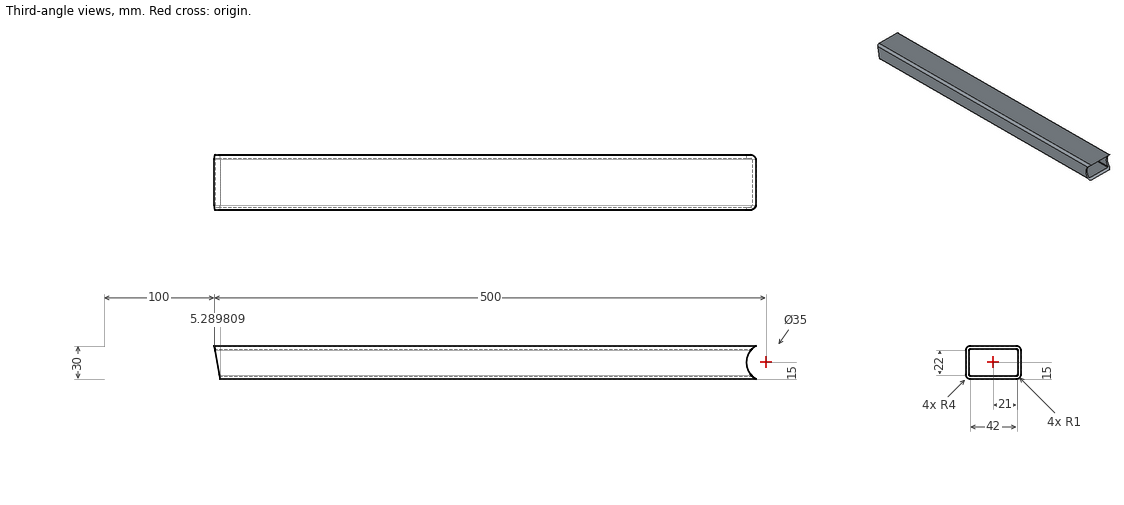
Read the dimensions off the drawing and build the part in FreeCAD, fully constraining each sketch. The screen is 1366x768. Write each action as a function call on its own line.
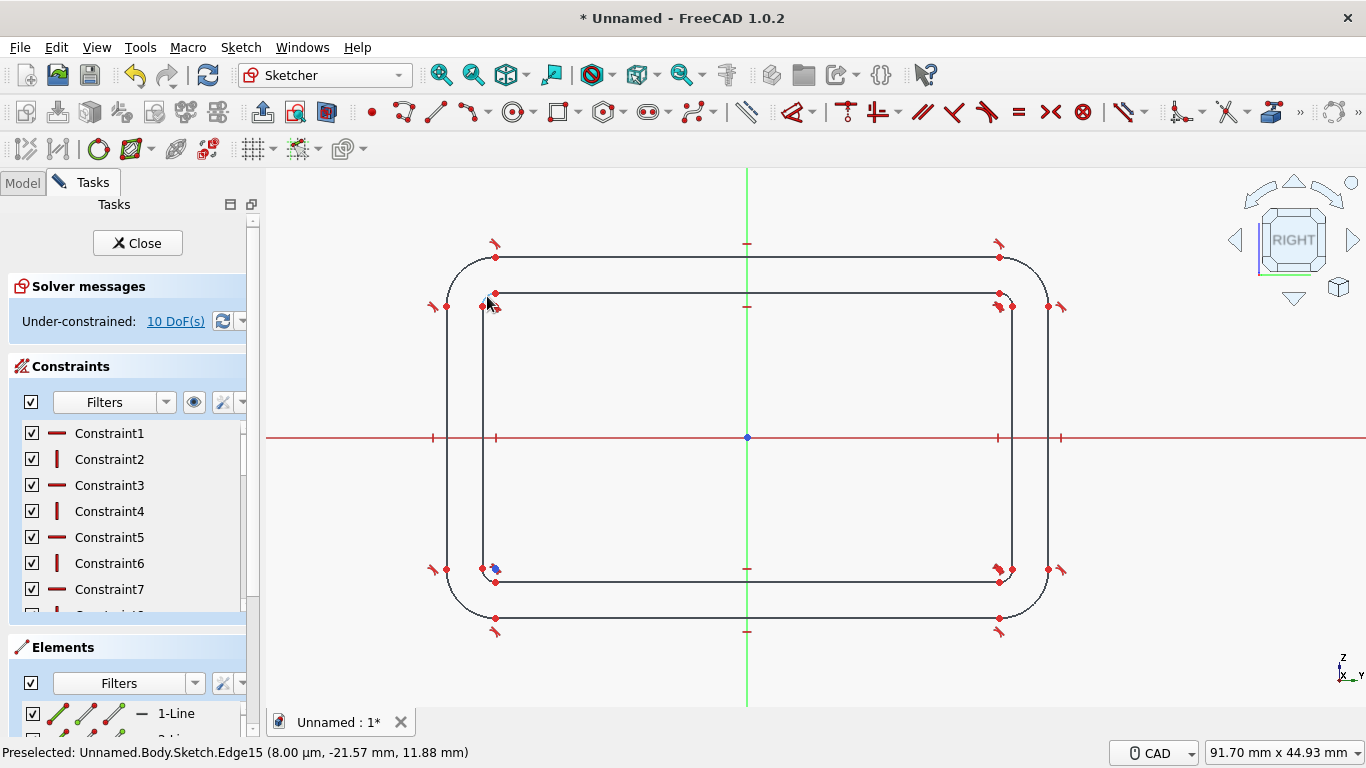
click(452, 591)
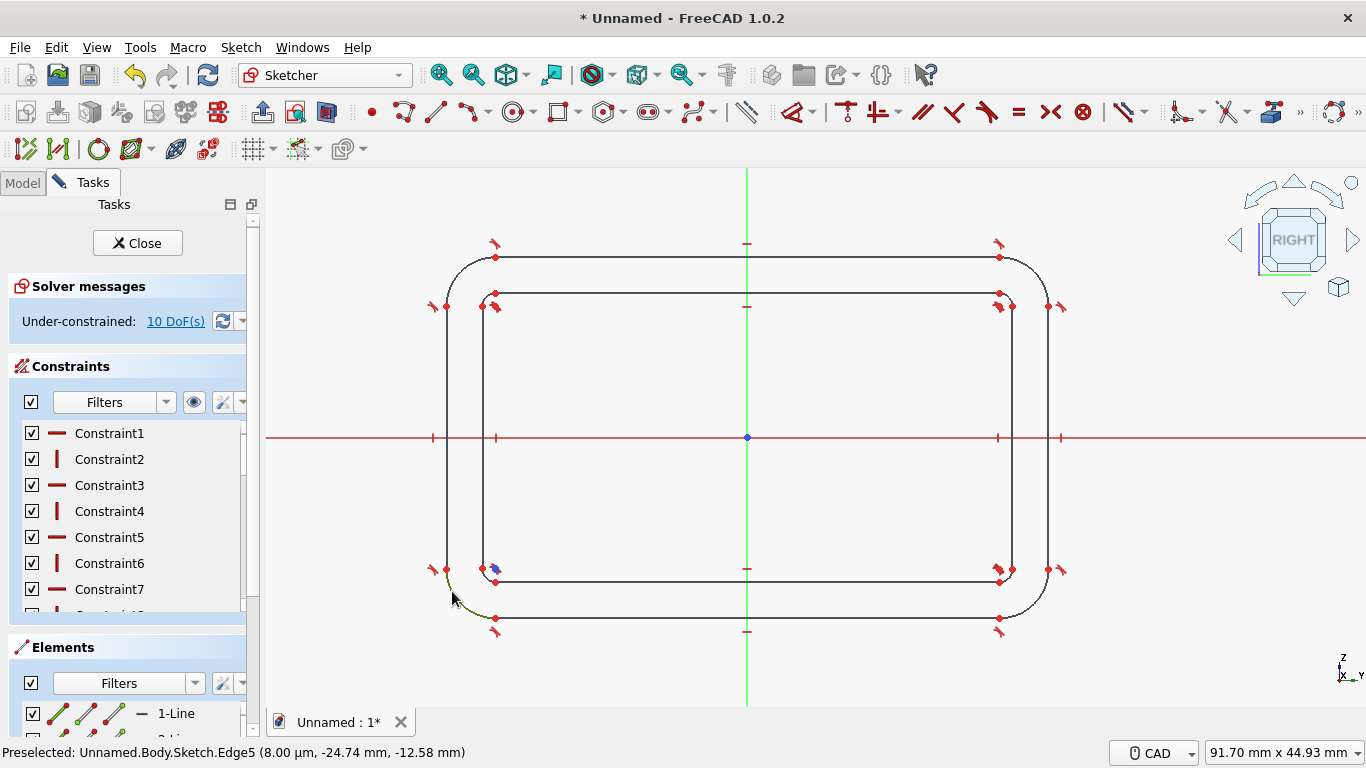
click(473, 263)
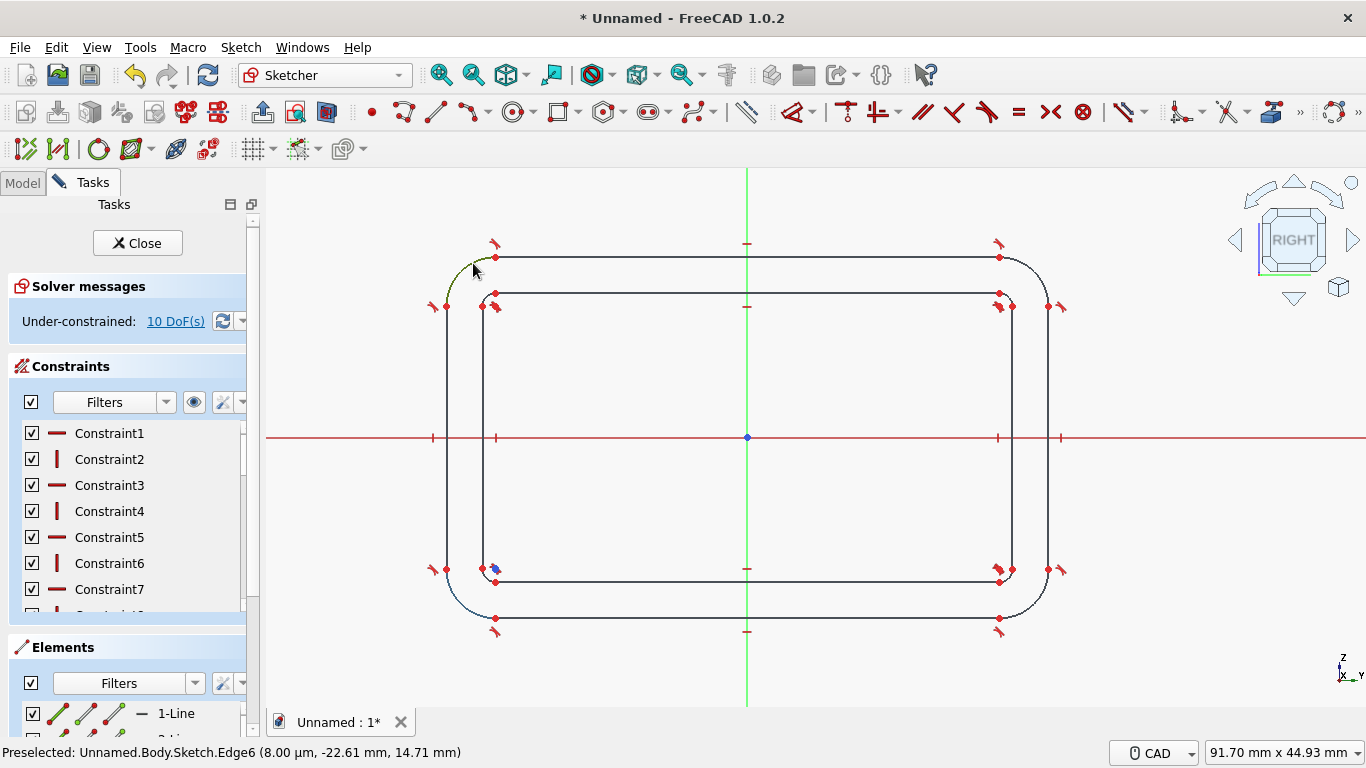
click(1043, 284)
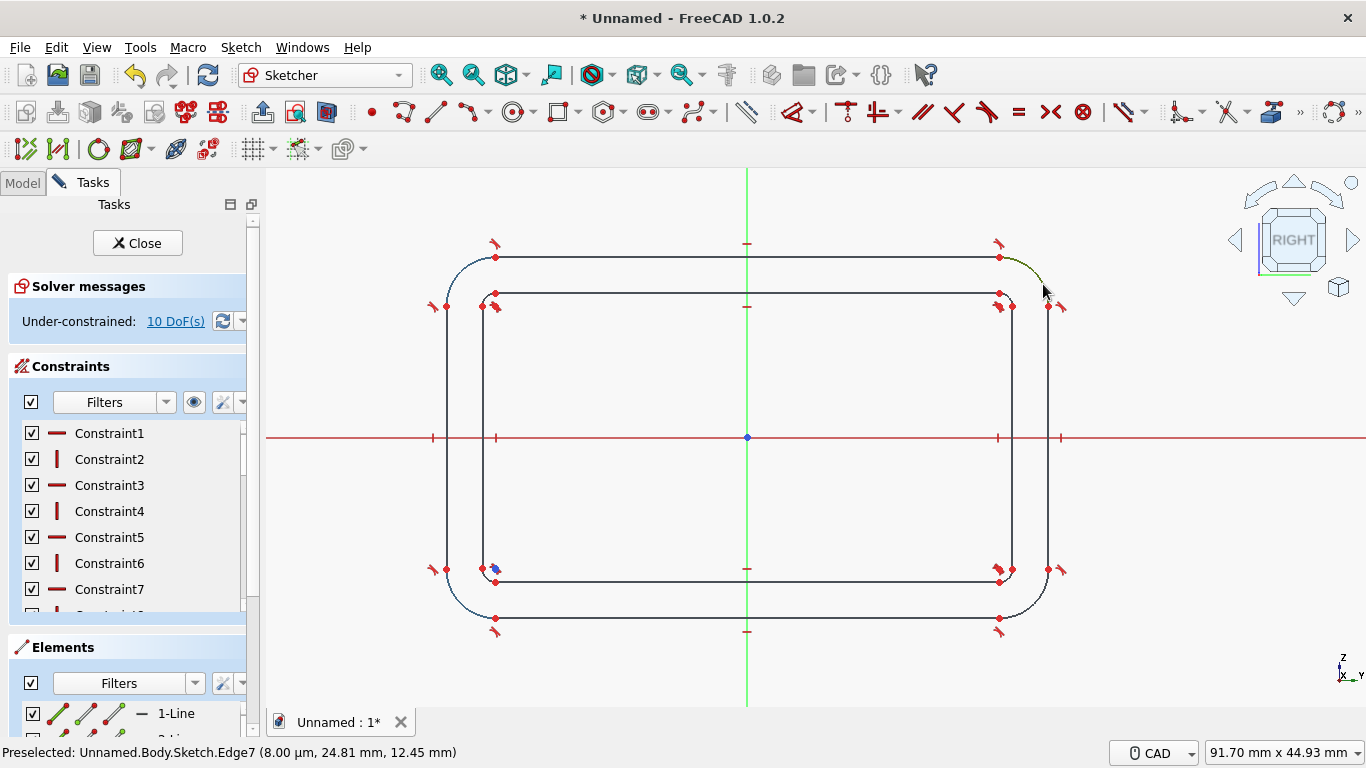
click(1022, 613)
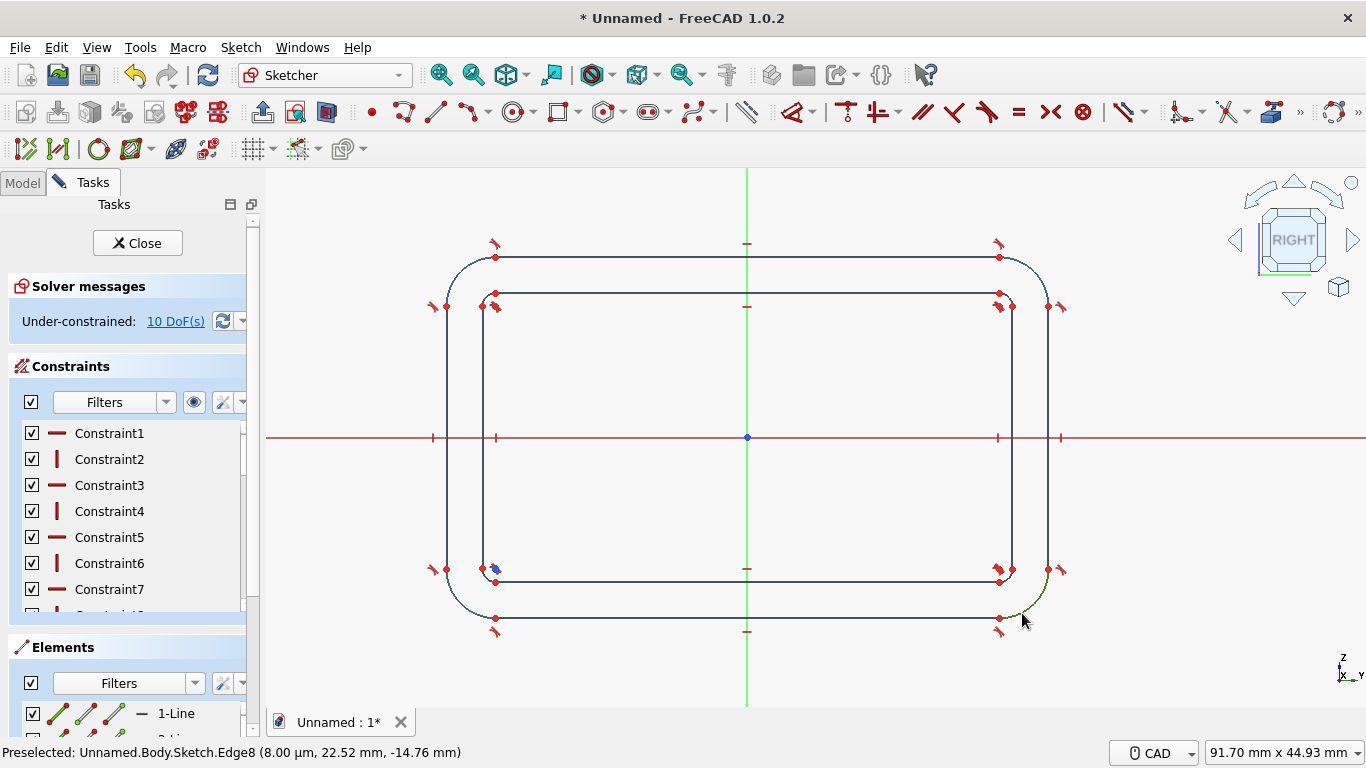
key(e)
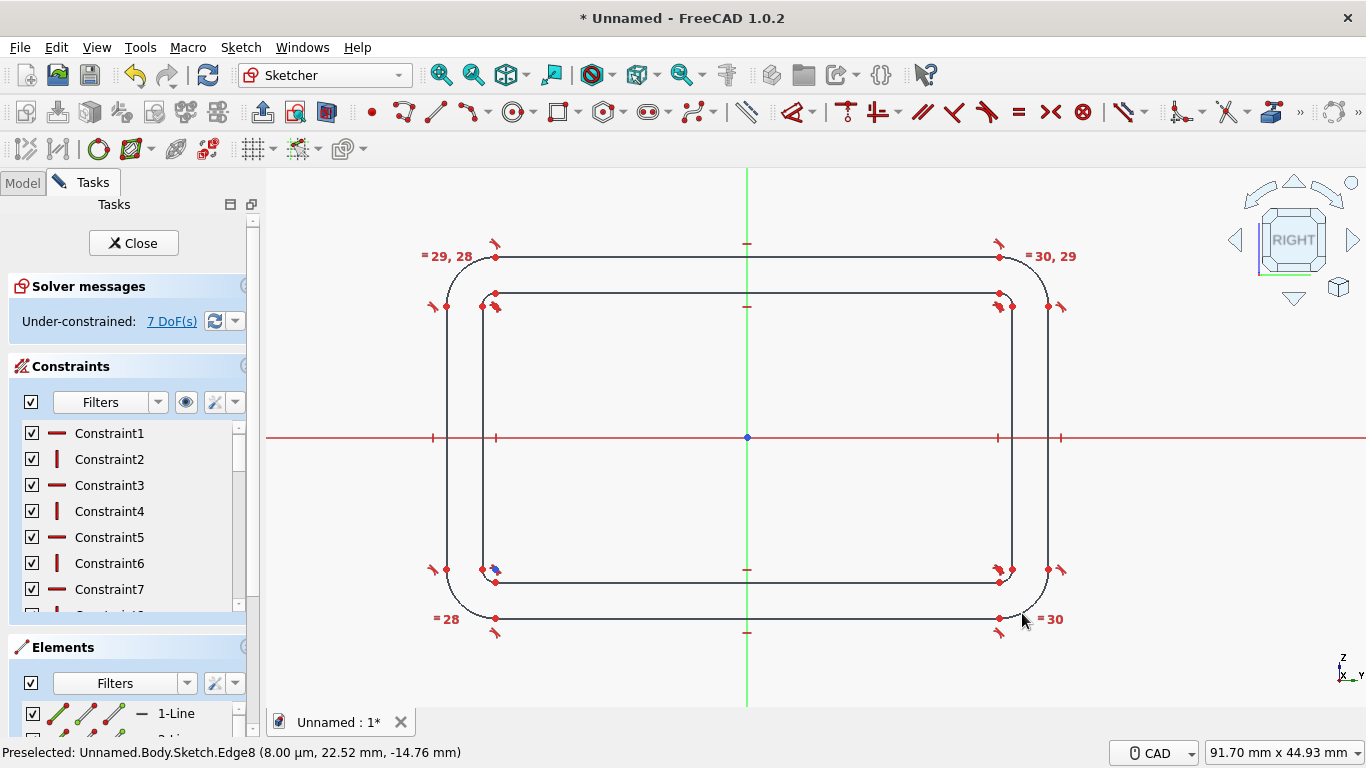
scroll(1009, 579, up, 2)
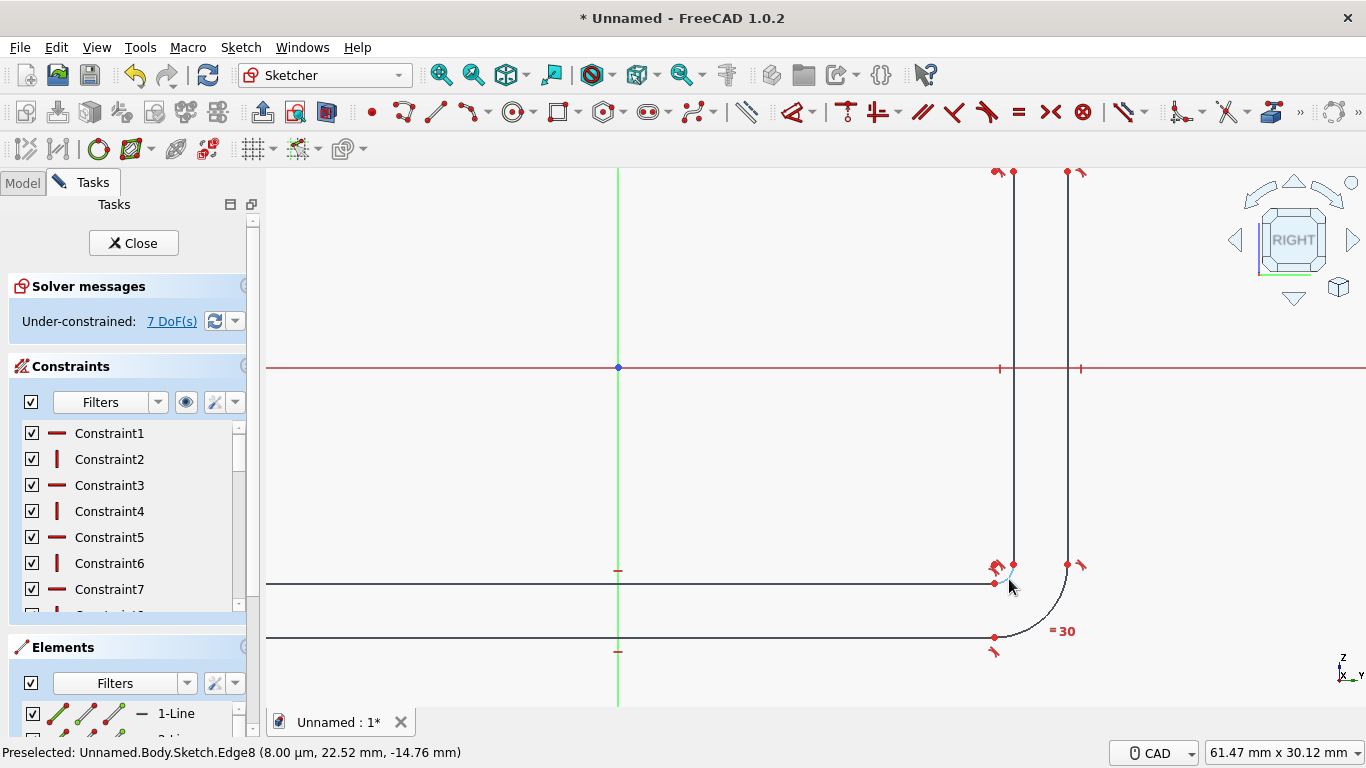
click(1008, 578)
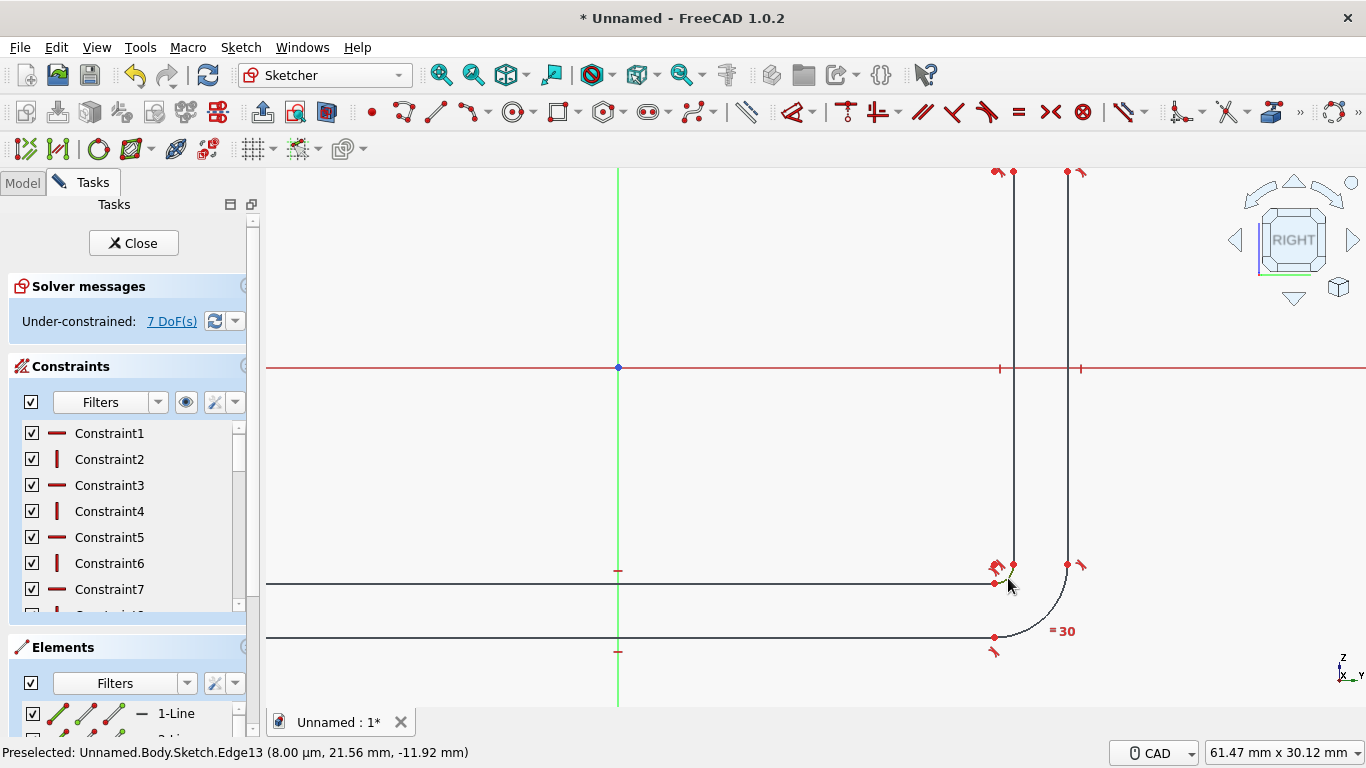
scroll(1010, 579, down, 2)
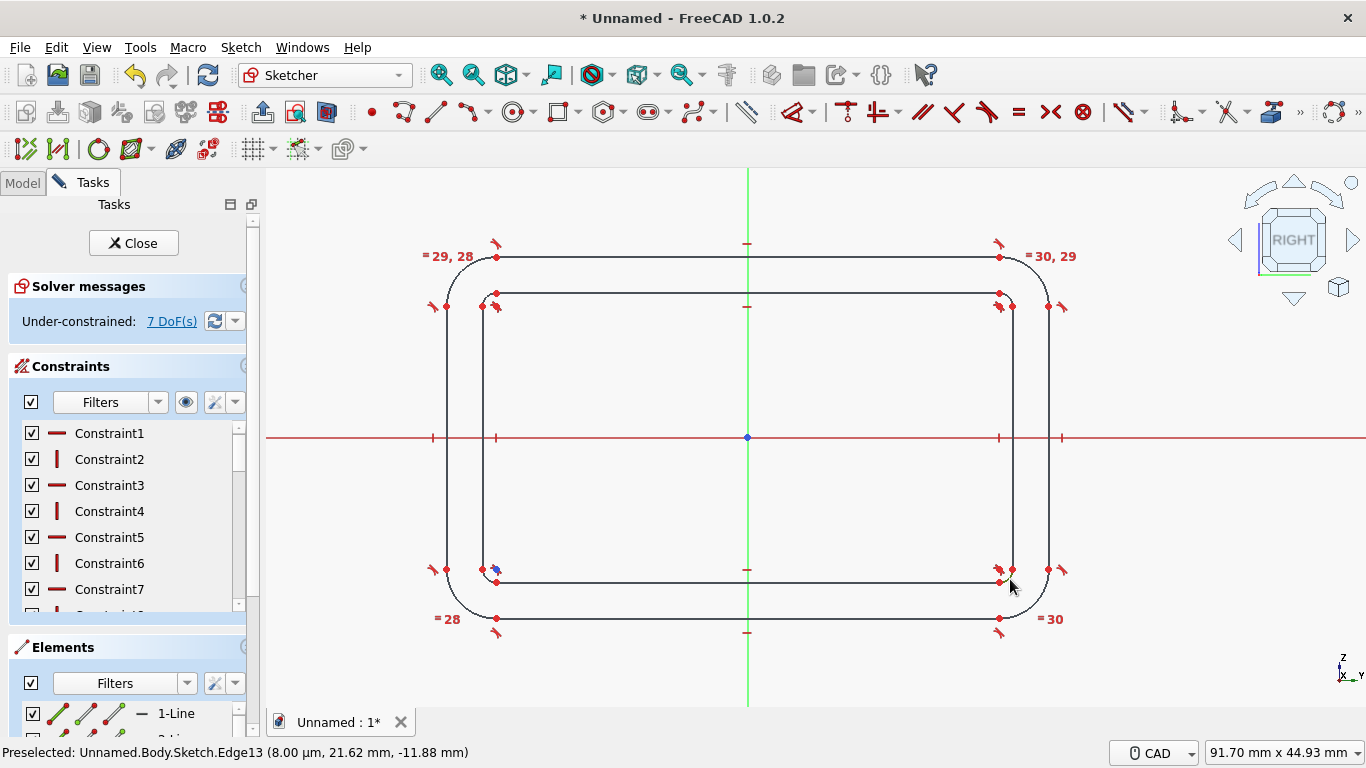
scroll(484, 575, up, 4)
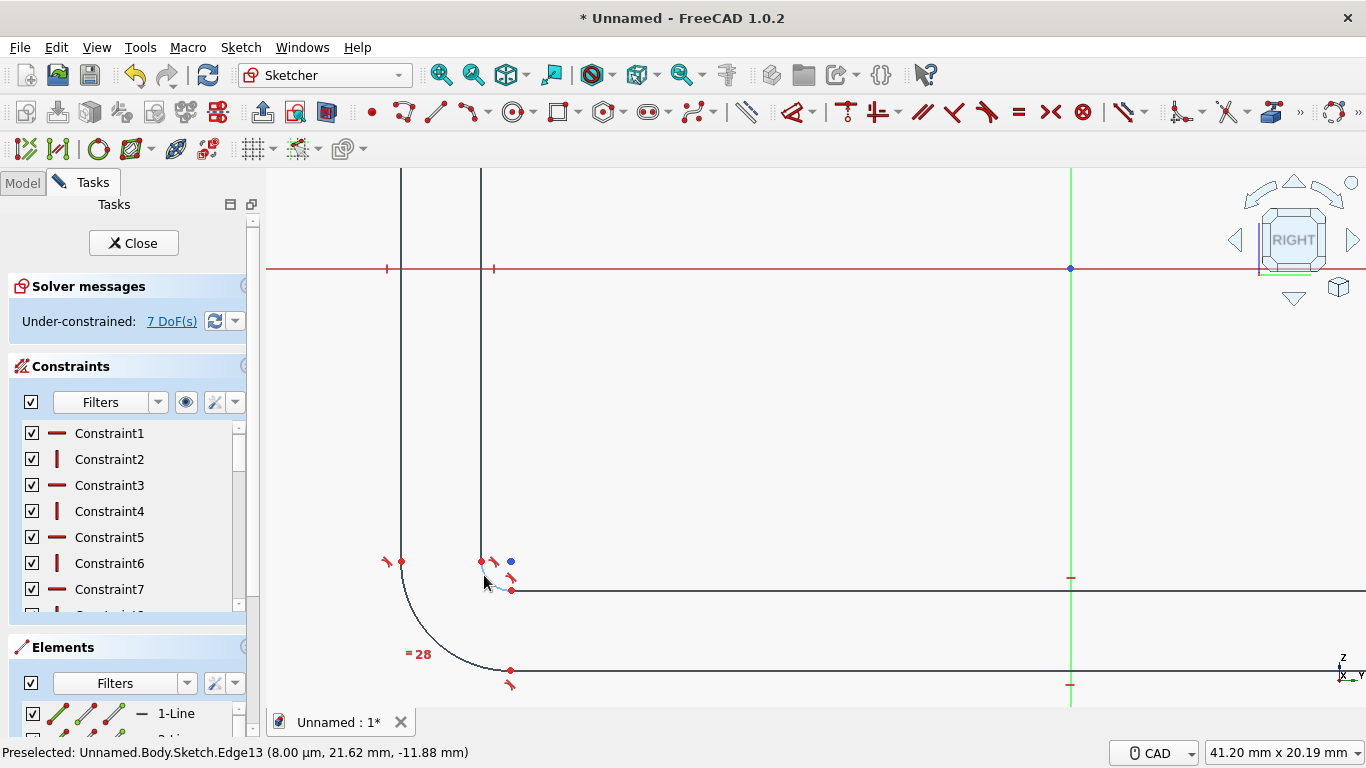
click(485, 575)